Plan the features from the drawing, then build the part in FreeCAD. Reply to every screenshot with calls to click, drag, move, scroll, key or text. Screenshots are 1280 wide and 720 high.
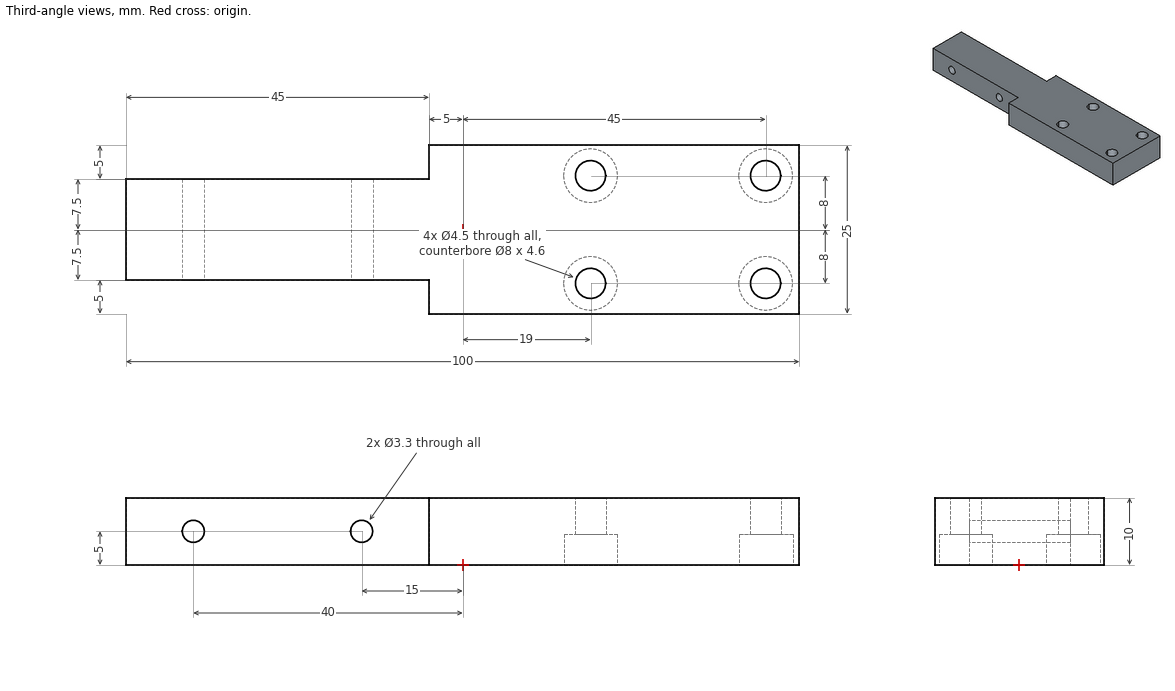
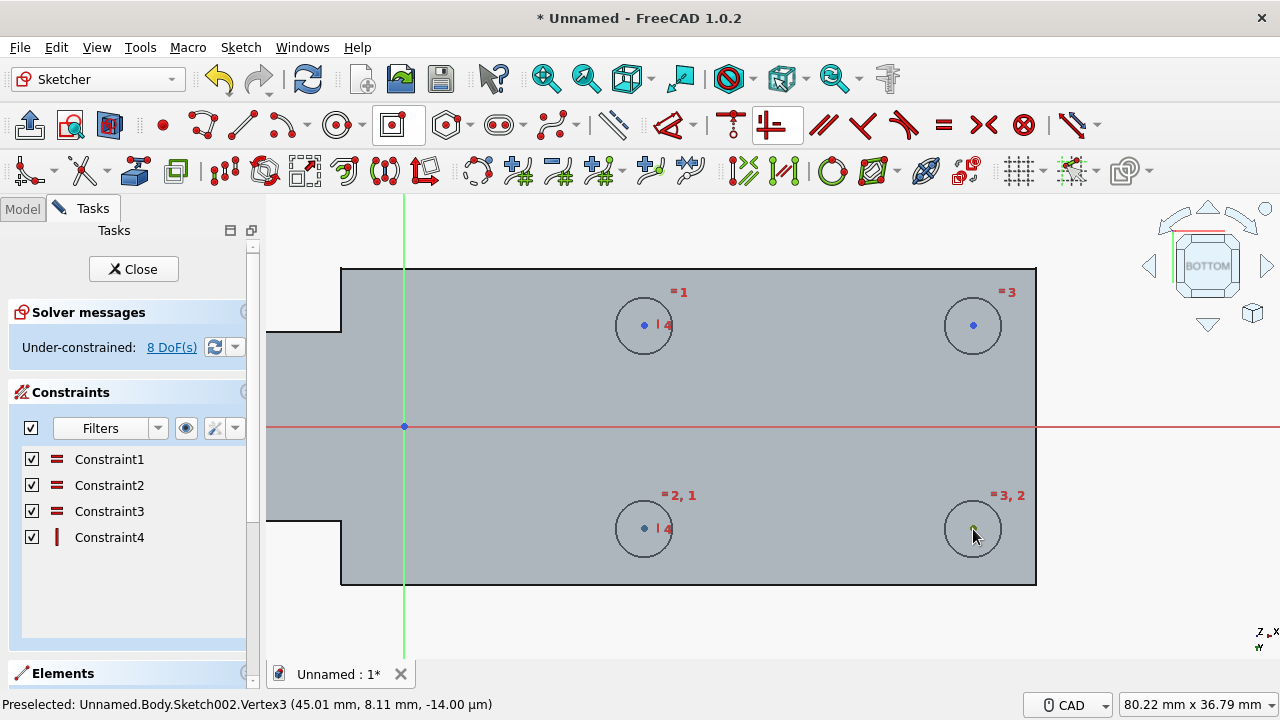
click(798, 126)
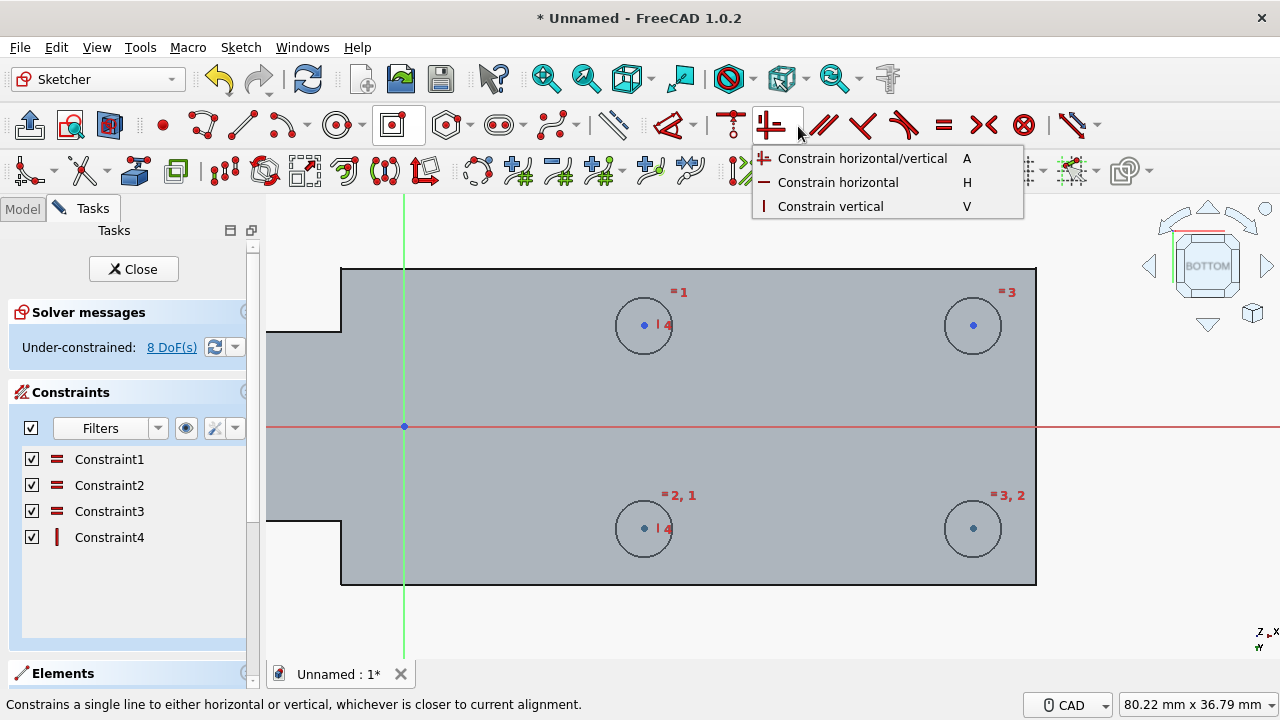
click(888, 182)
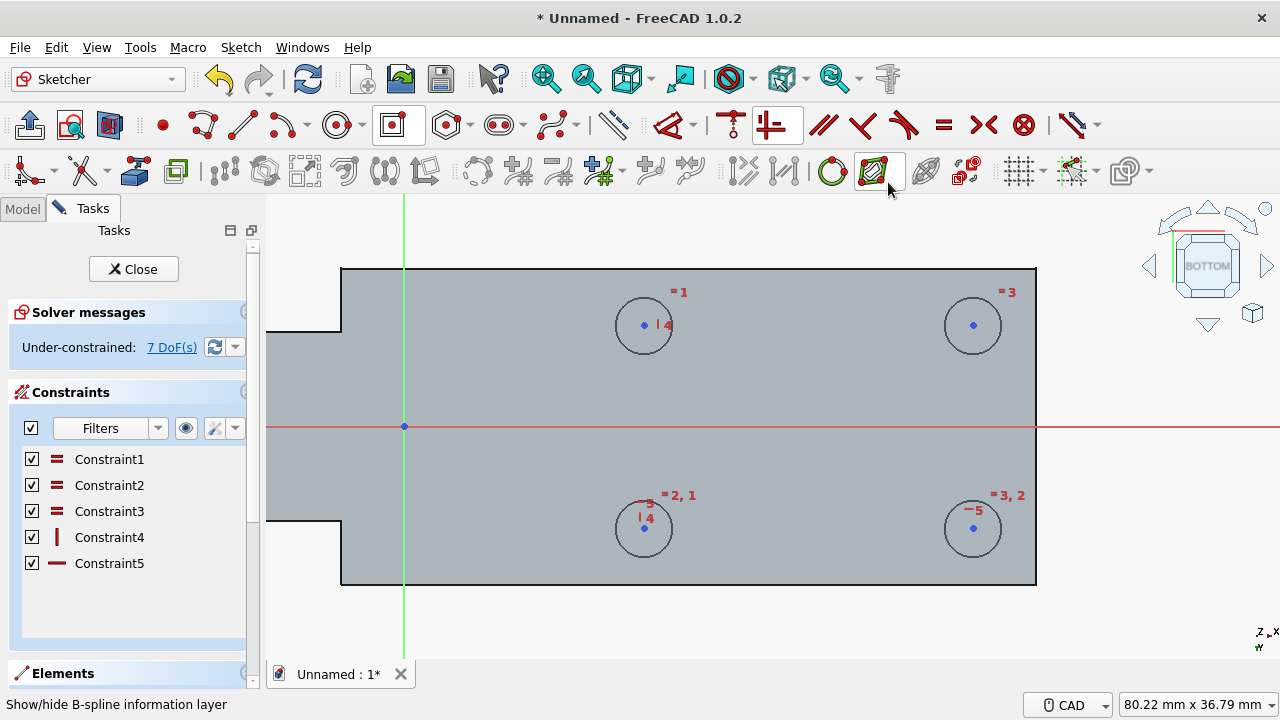
click(973, 529)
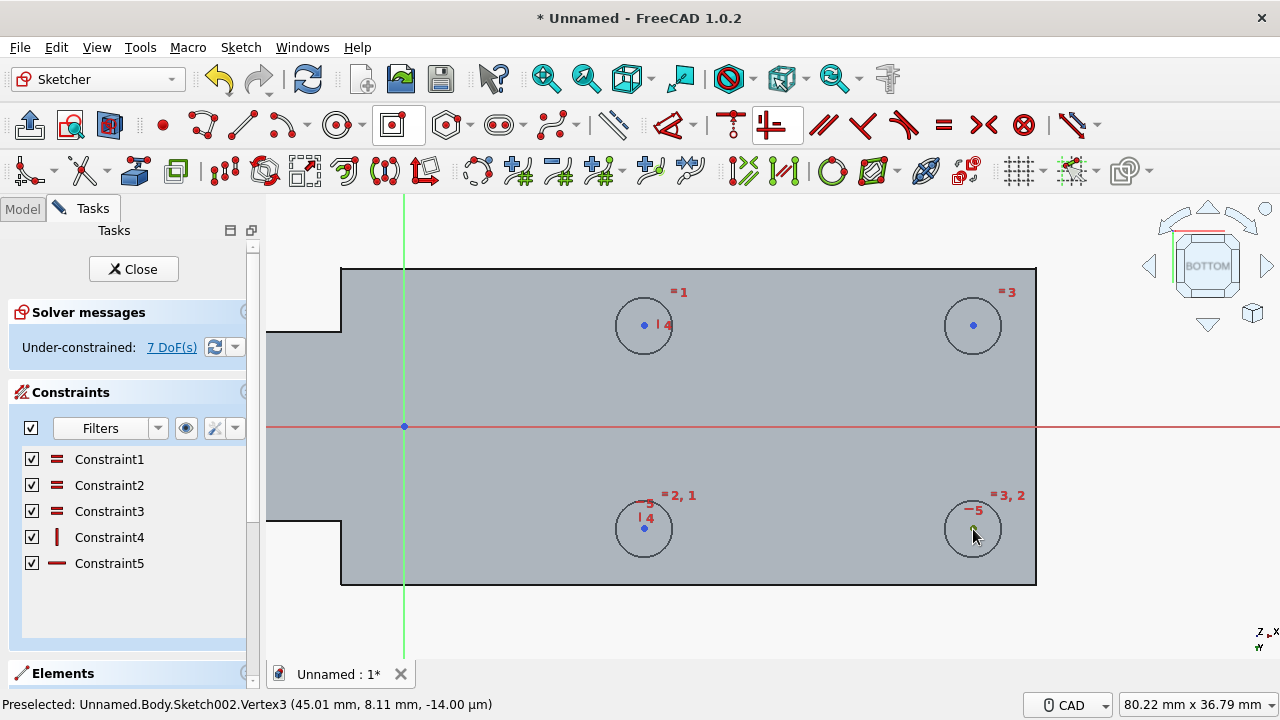
click(973, 326)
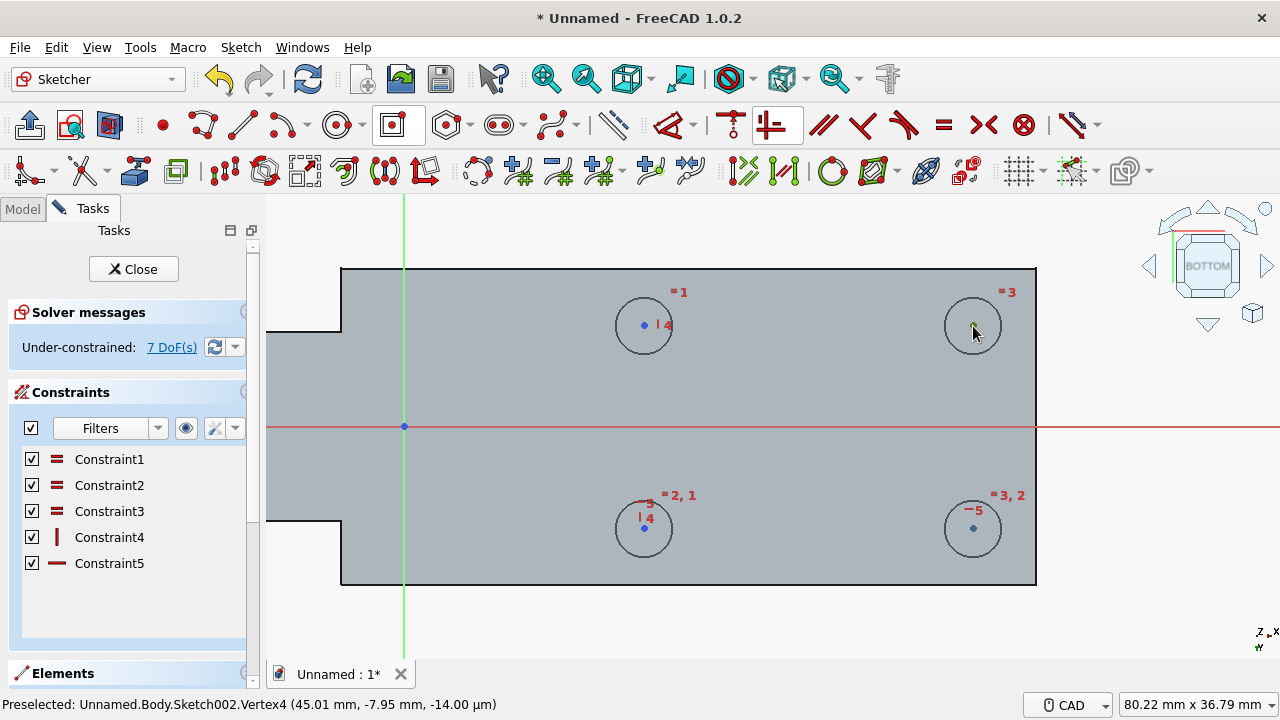
click(798, 126)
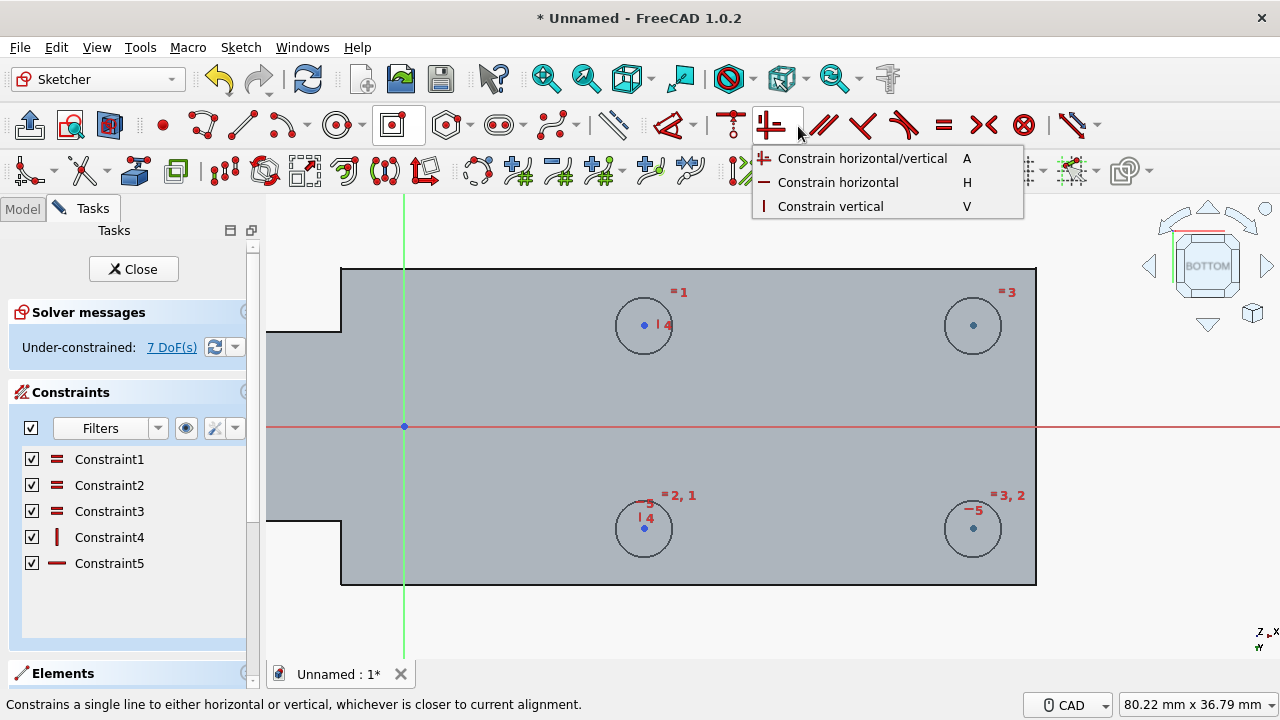
click(888, 206)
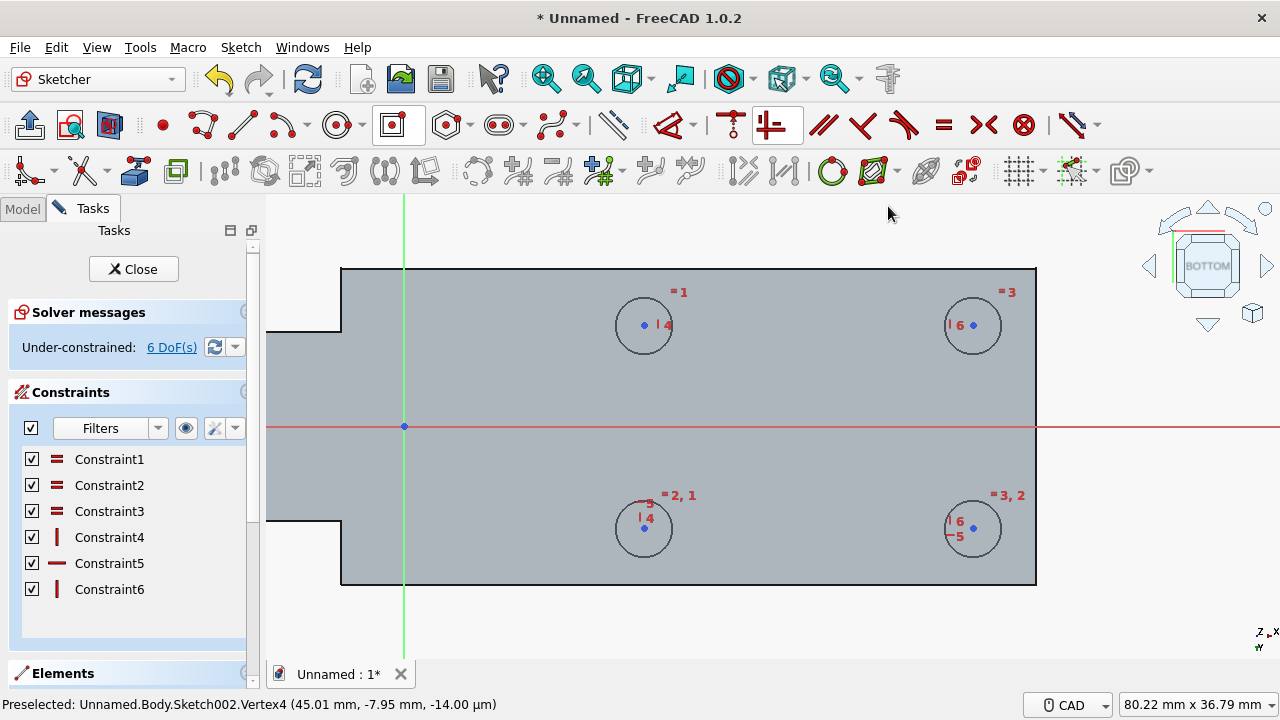
click(644, 326)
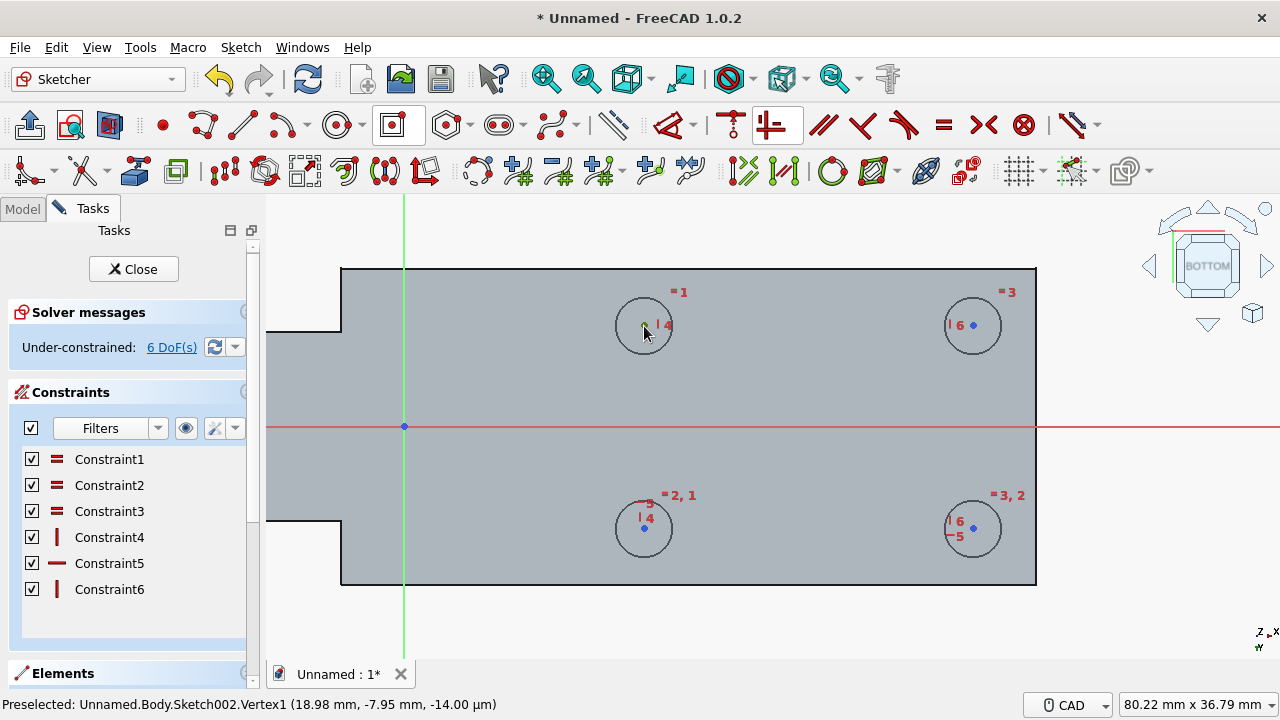
click(973, 326)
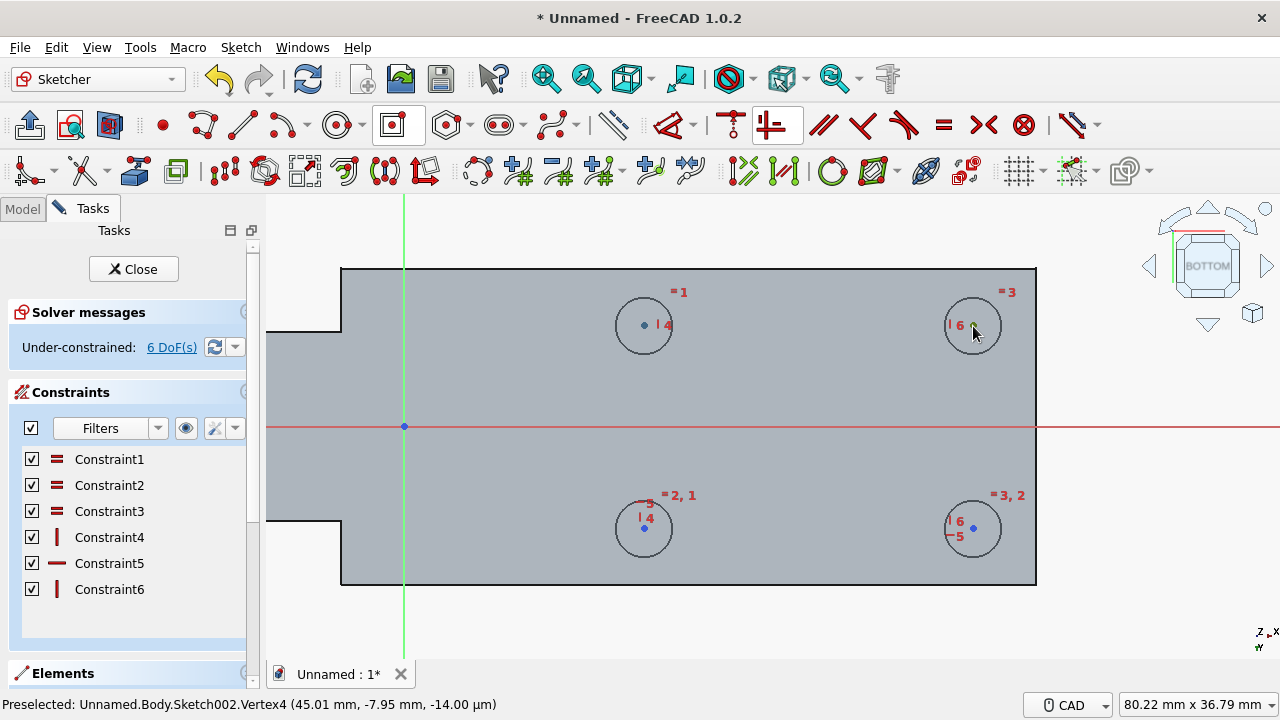
key(h)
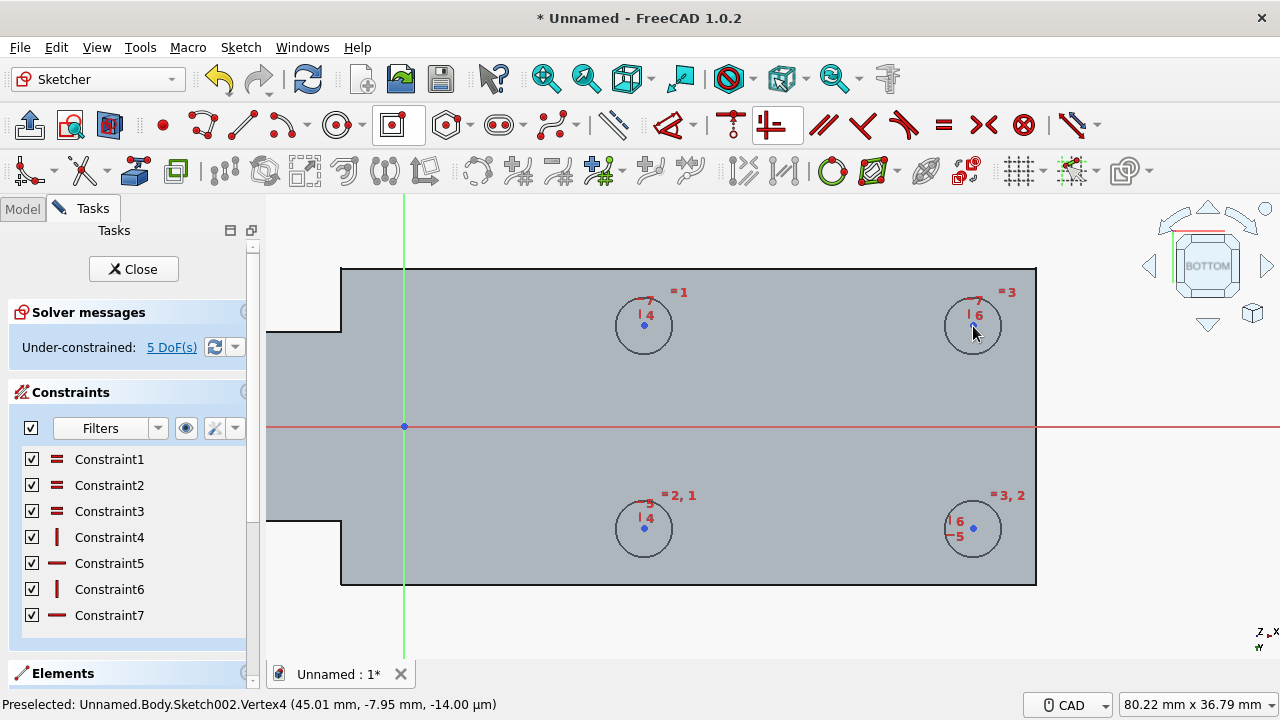
click(668, 126)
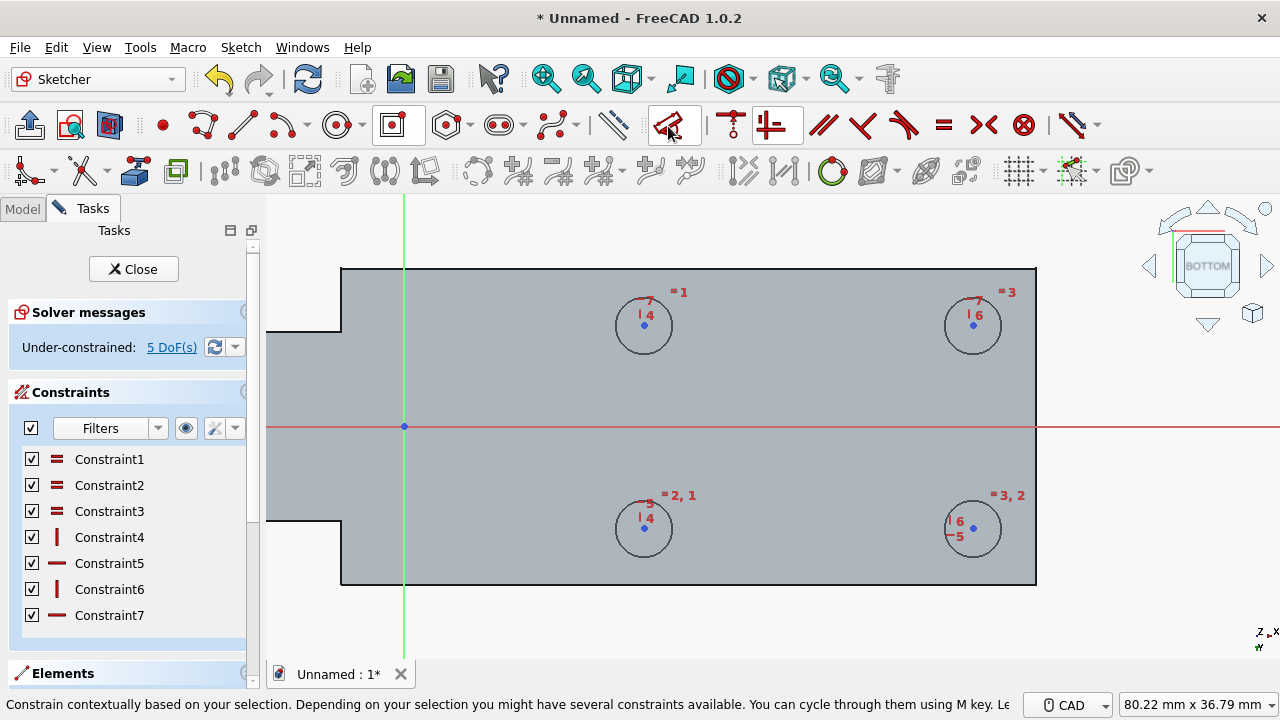
click(664, 306)
click(687, 283)